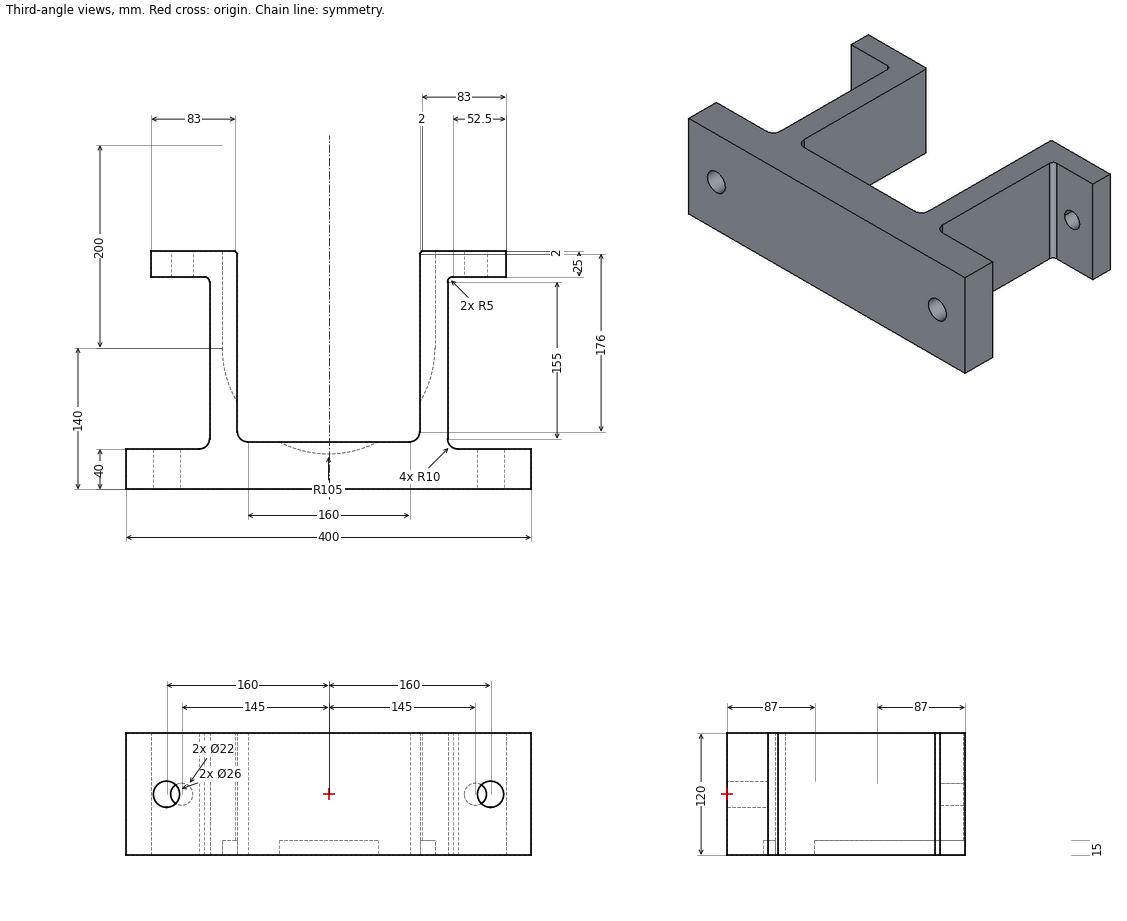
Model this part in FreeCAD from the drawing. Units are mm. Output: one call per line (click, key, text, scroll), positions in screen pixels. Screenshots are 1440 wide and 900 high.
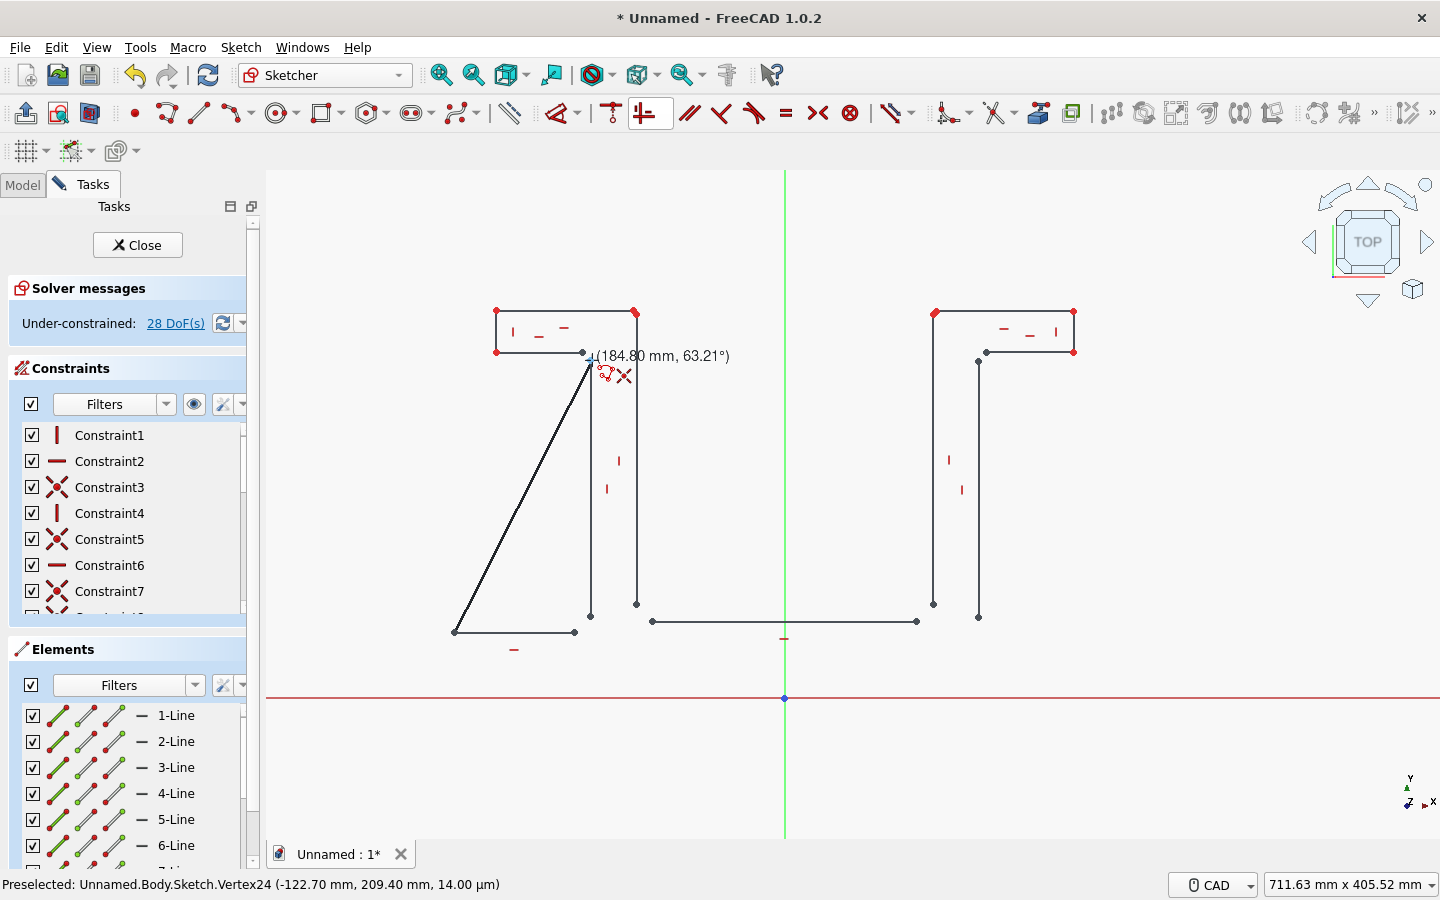
click(455, 698)
click(1115, 689)
click(1115, 632)
click(995, 632)
right_click(995, 632)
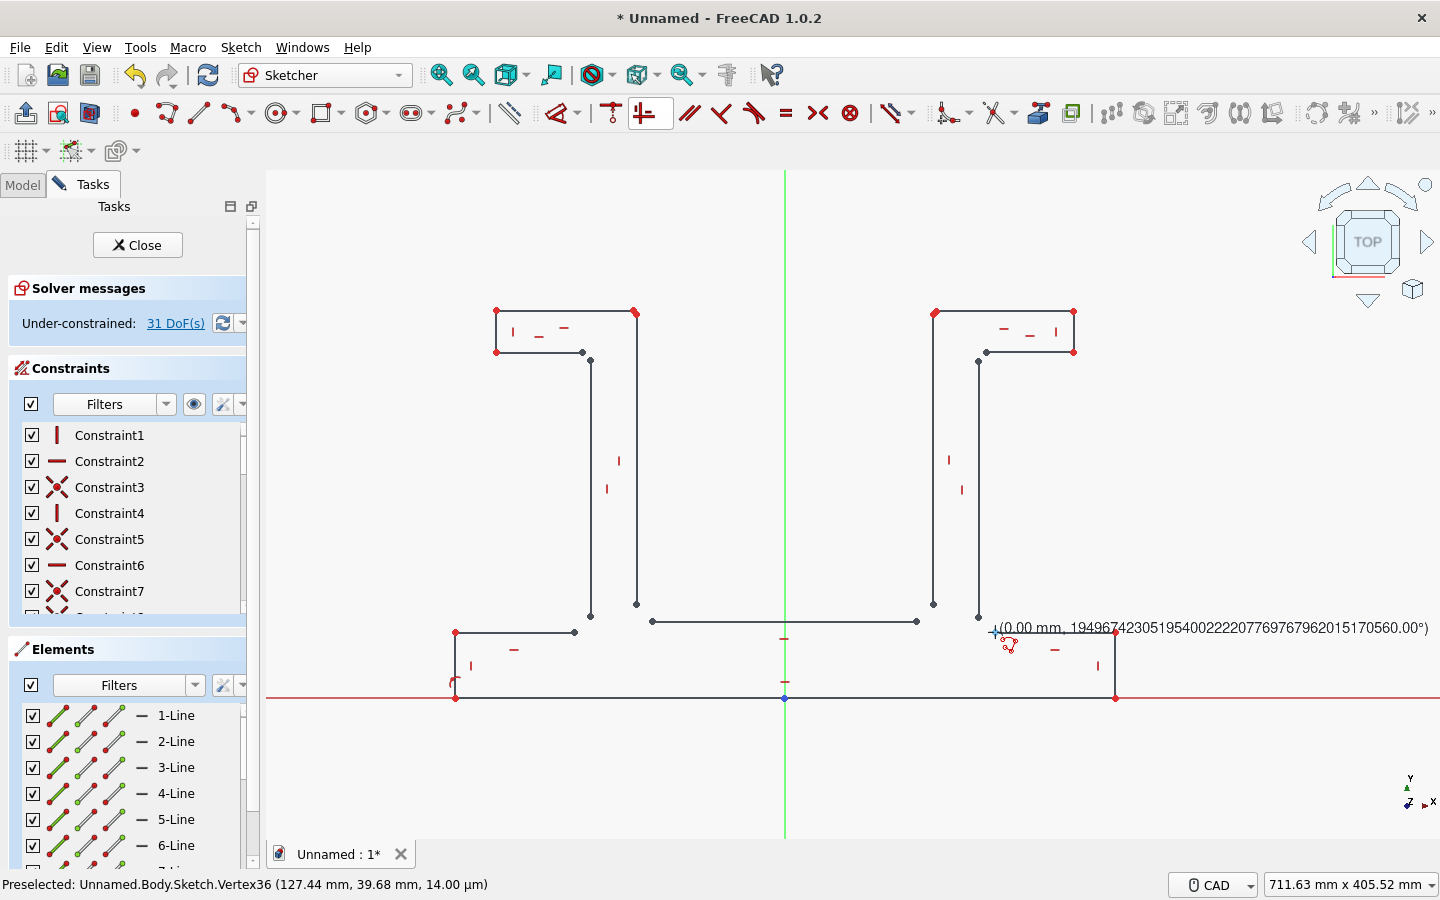
click(232, 114)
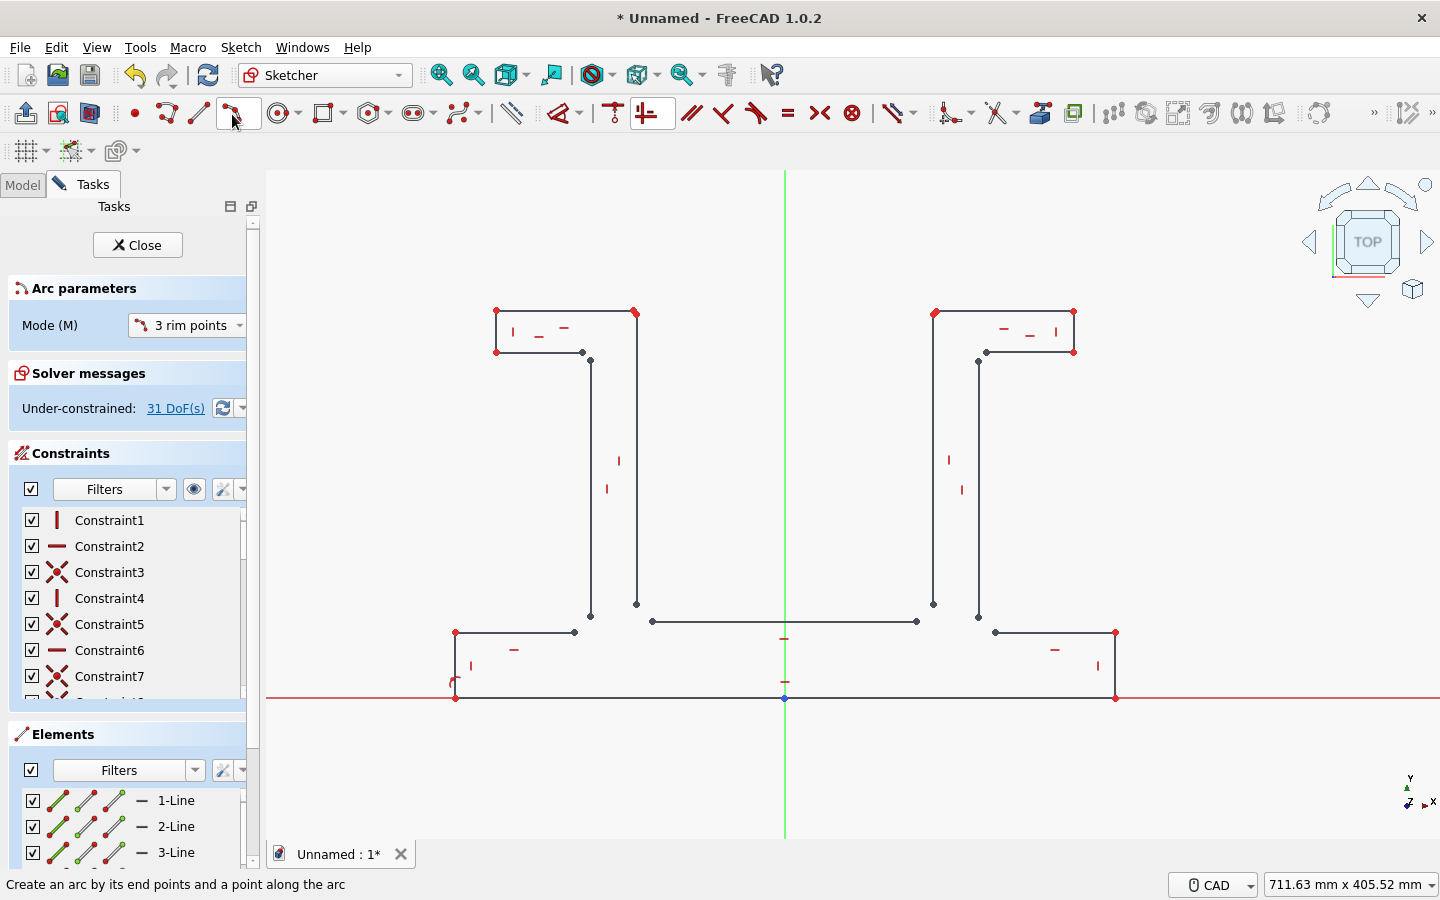
scroll(979, 360, up, 2)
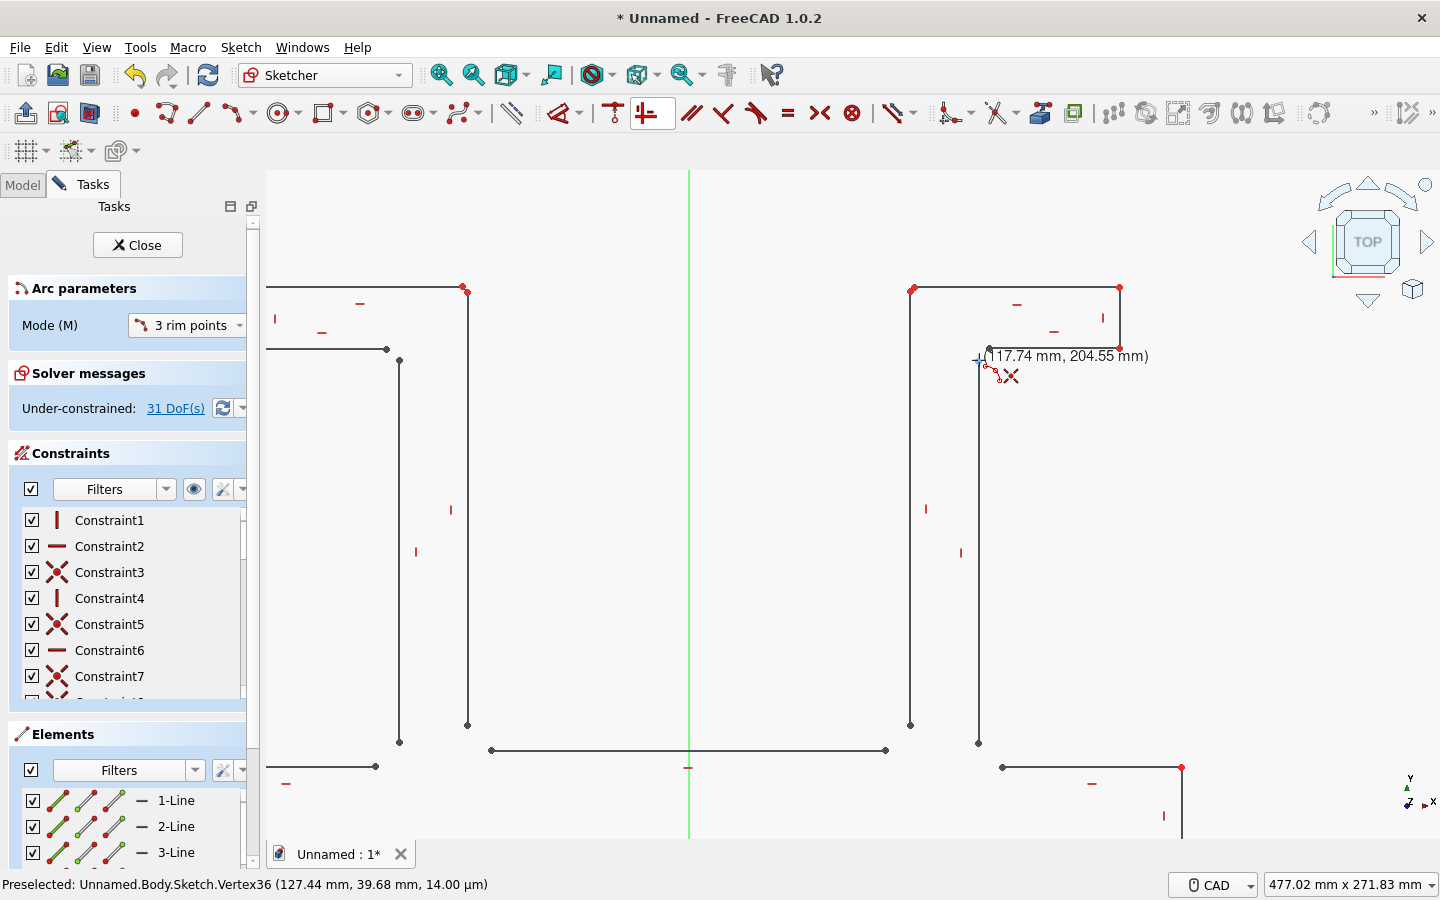
click(979, 362)
click(990, 348)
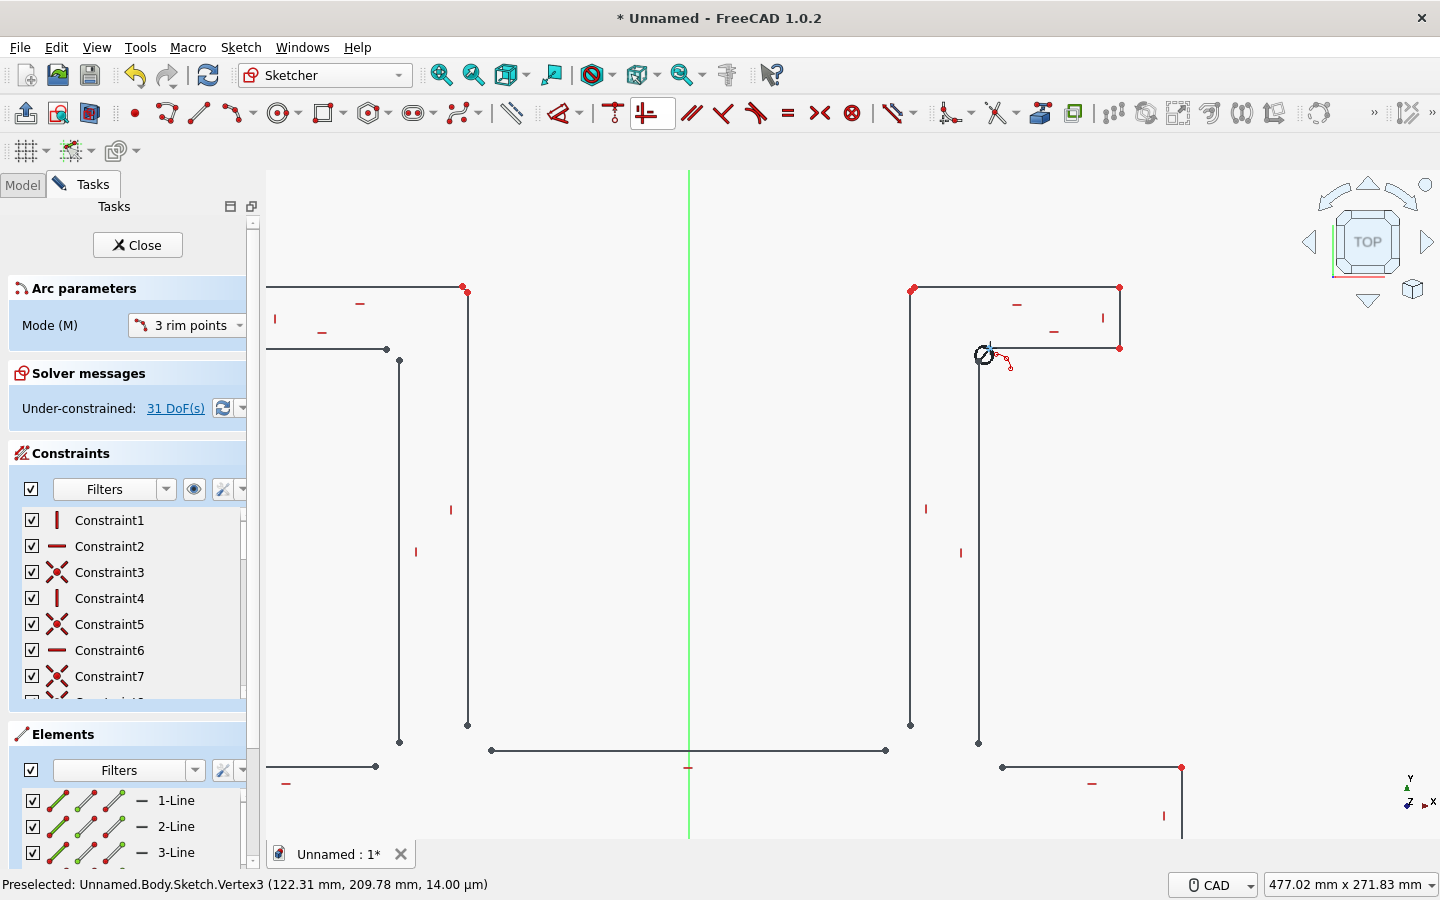
scroll(982, 352, up, 8)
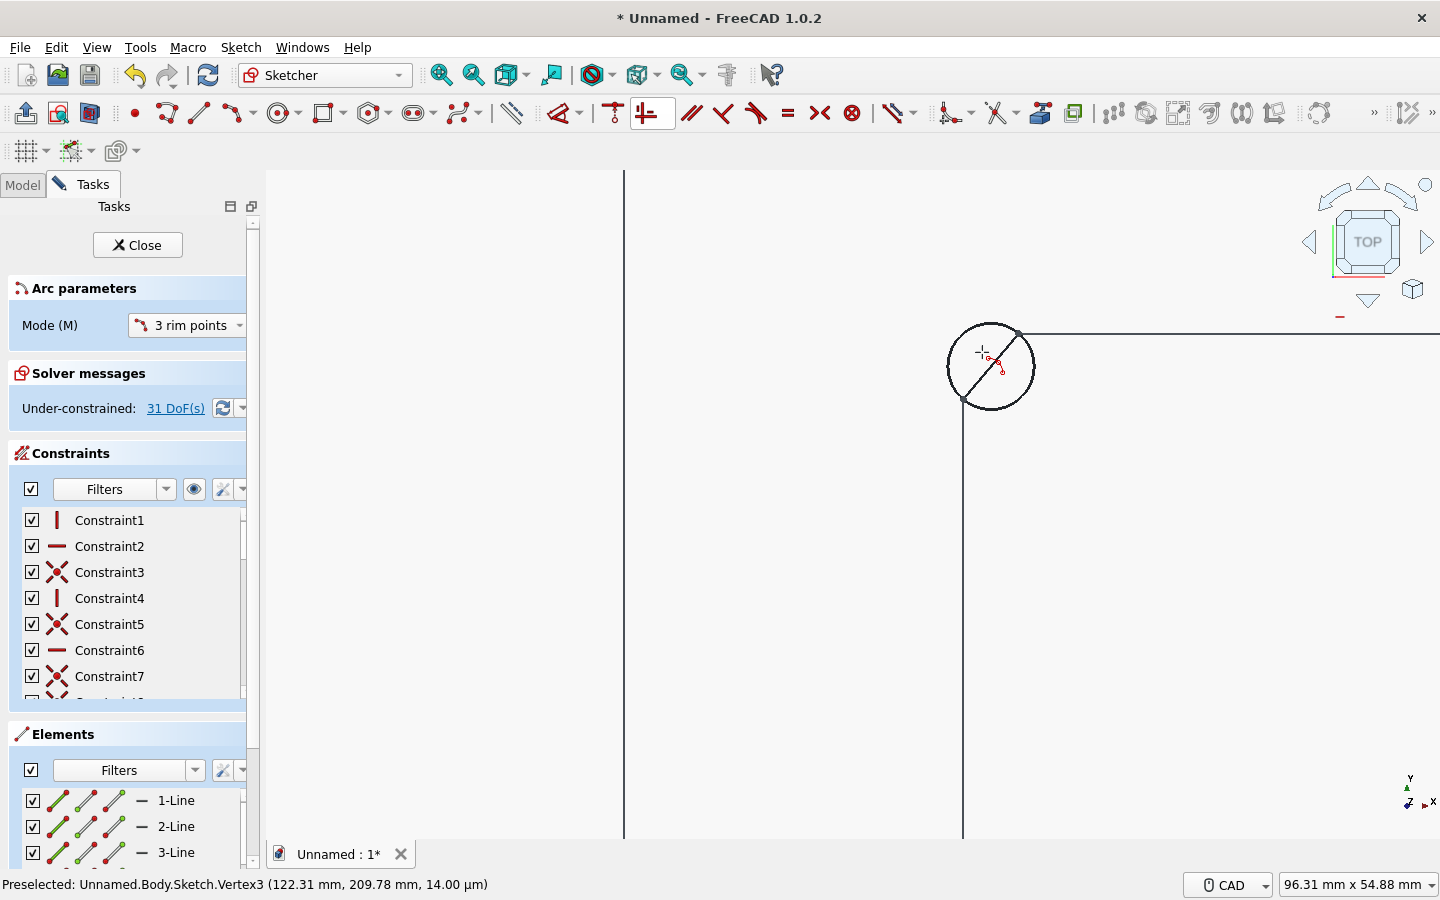
click(978, 349)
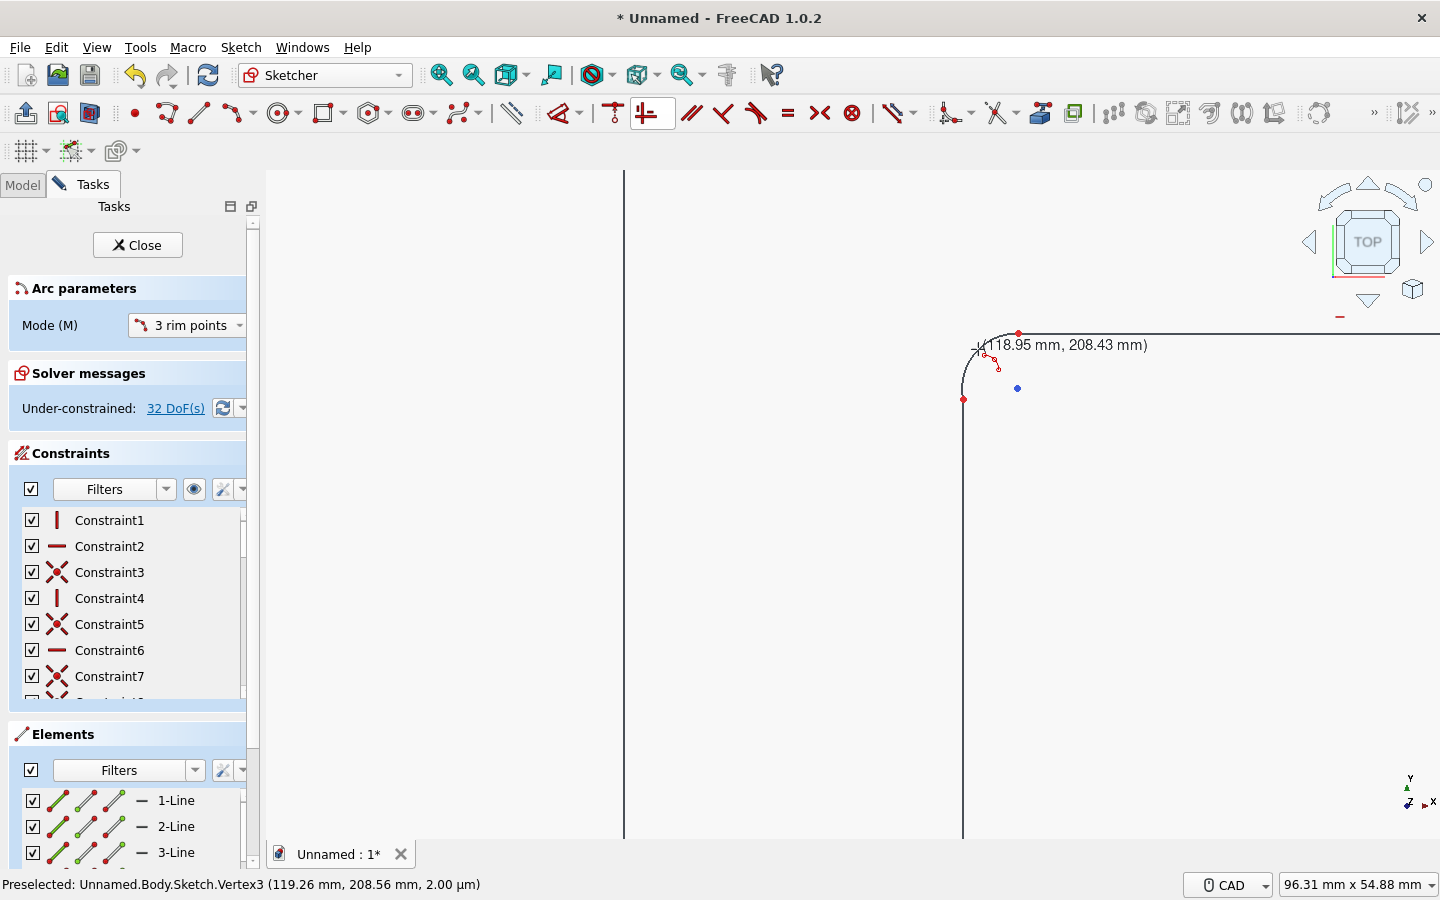
scroll(981, 355, down, 10)